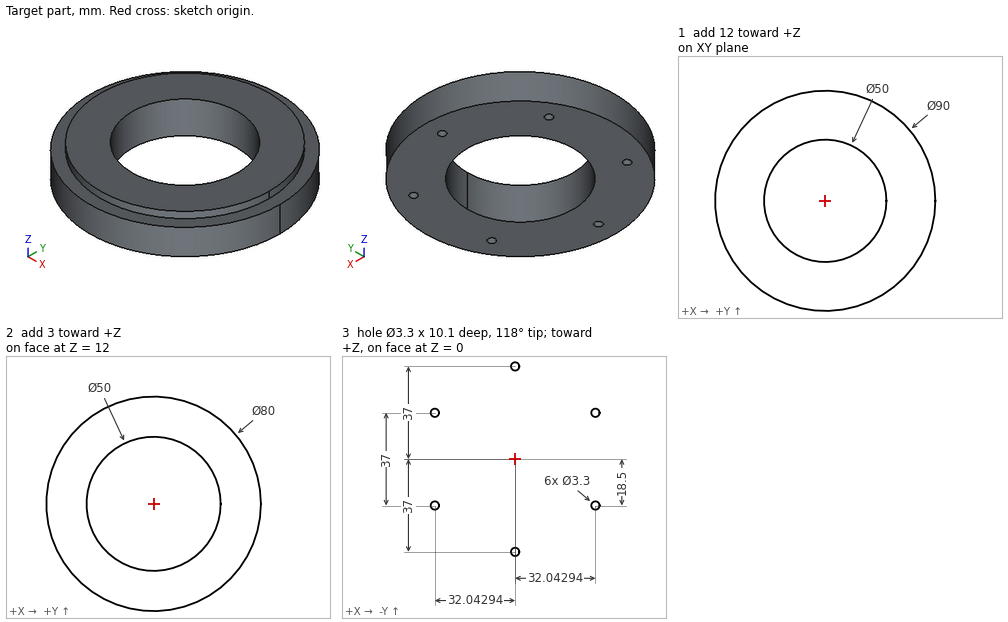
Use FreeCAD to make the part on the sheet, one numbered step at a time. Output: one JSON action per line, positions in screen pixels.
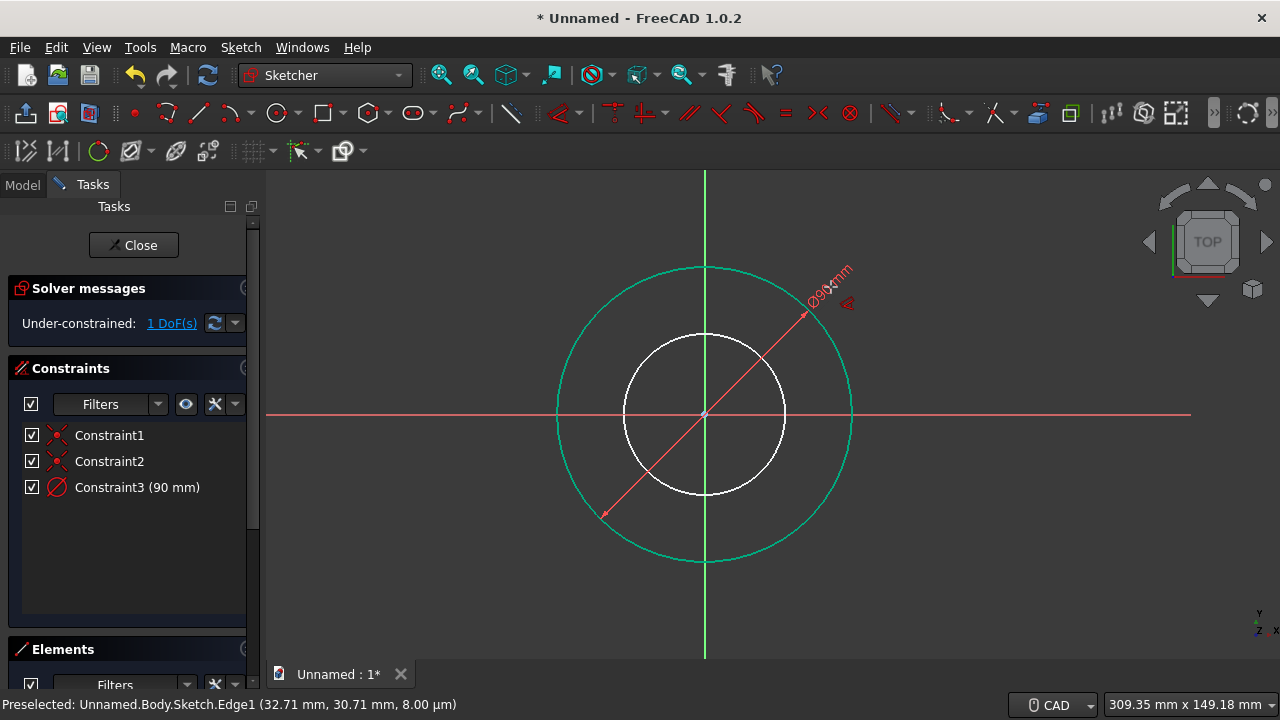
{"action": "left_click", "coordinate": [761, 357]}
{"action": "left_click", "coordinate": [783, 334]}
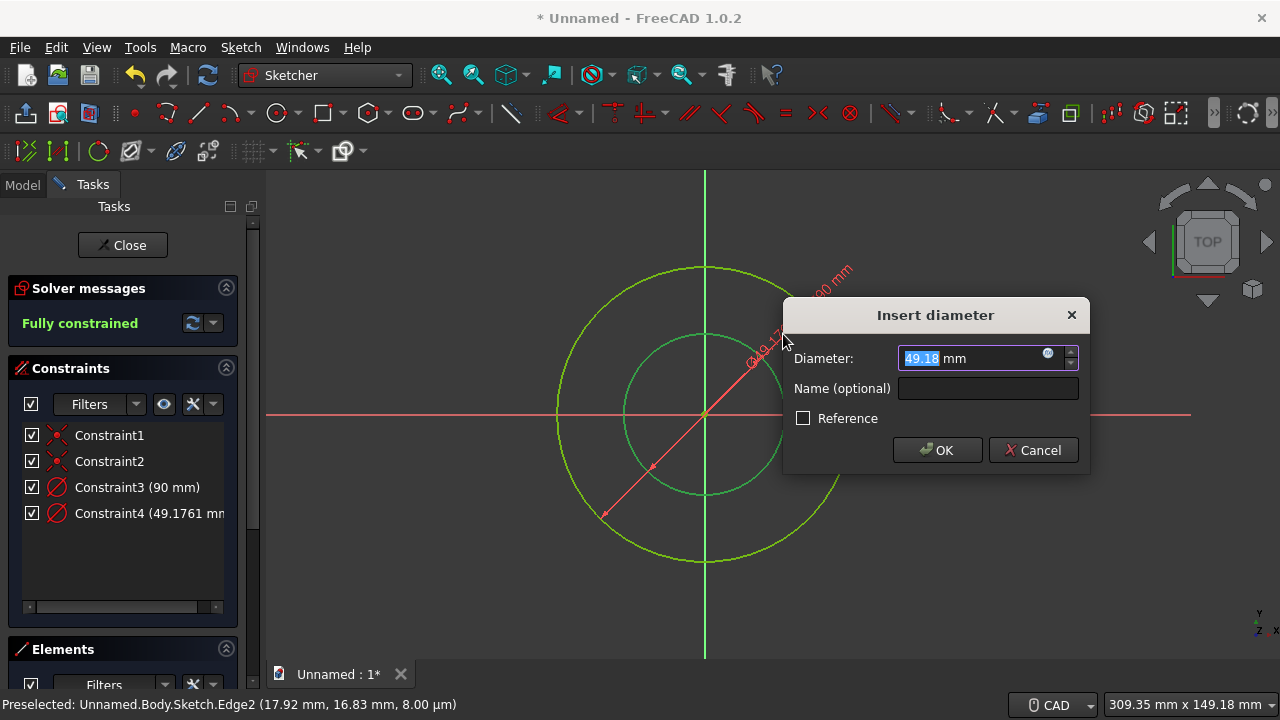
{"action": "type", "text": "50"}
{"action": "key", "text": "Return"}
{"action": "key", "text": "Escape"}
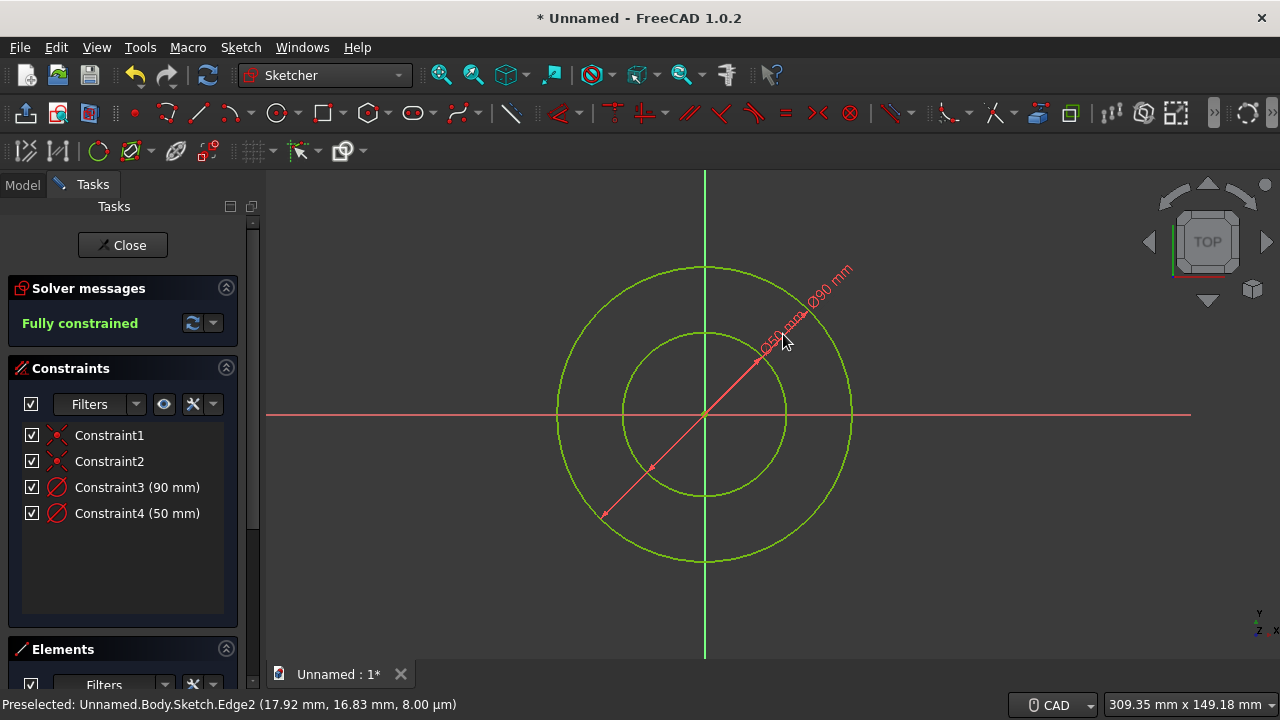
{"action": "left_click", "coordinate": [123, 245]}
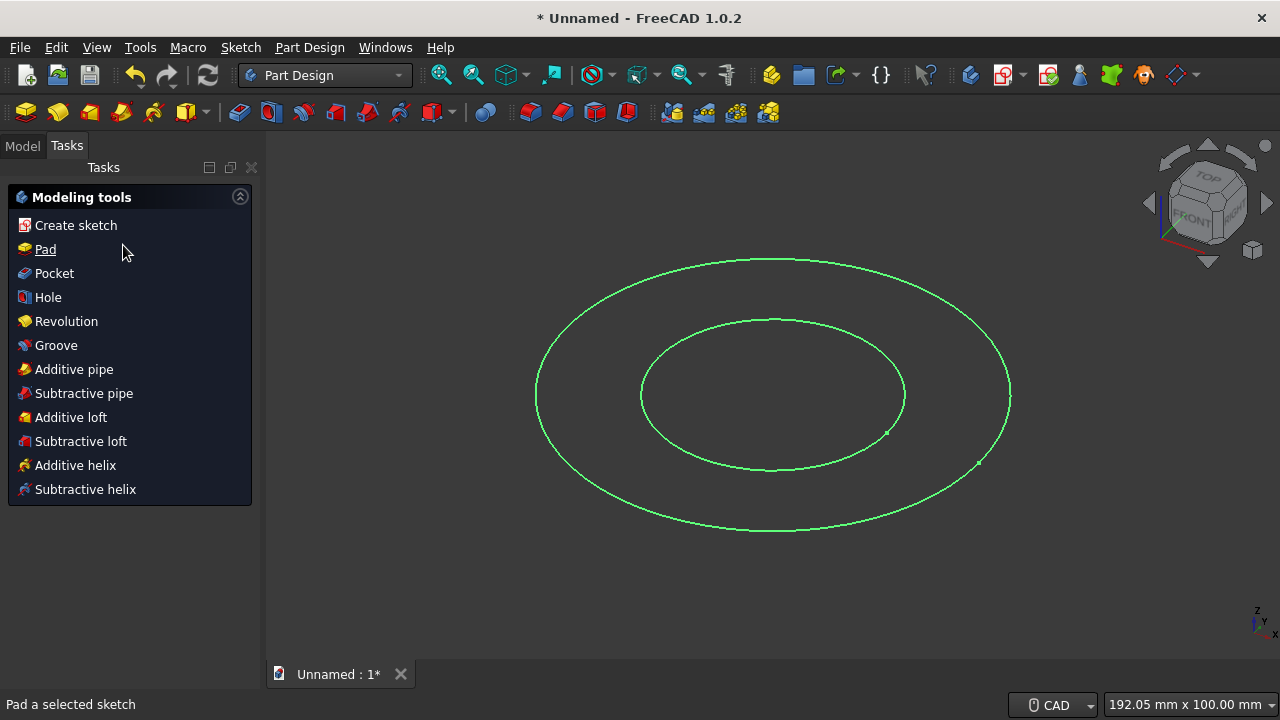
{"action": "left_click", "coordinate": [26, 112]}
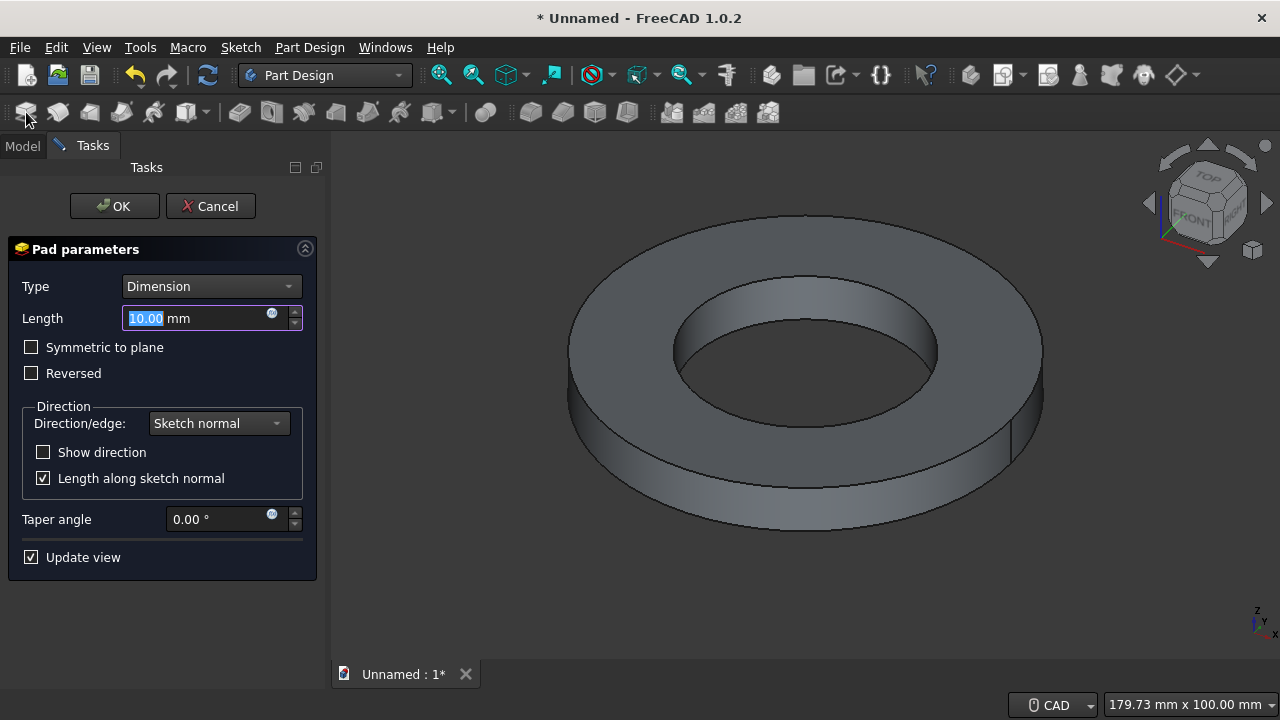
{"action": "type", "text": "12"}
{"action": "key", "text": "Tab"}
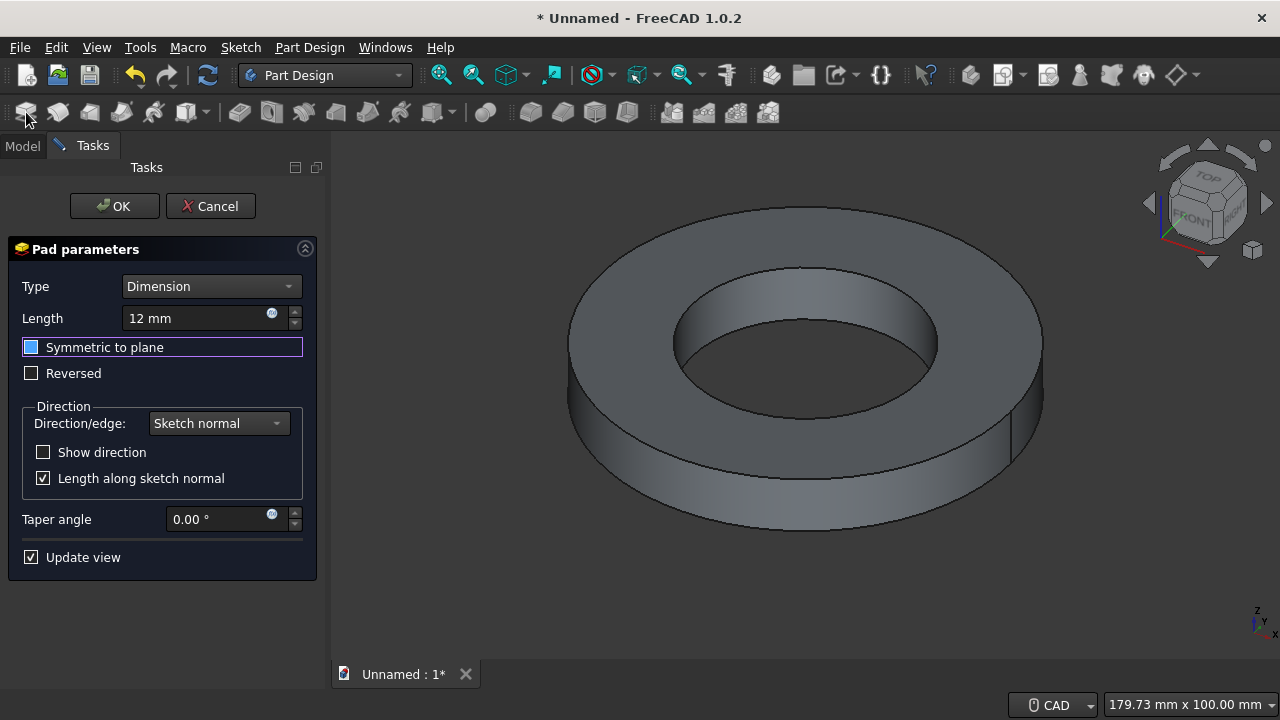
{"action": "left_click", "coordinate": [115, 206]}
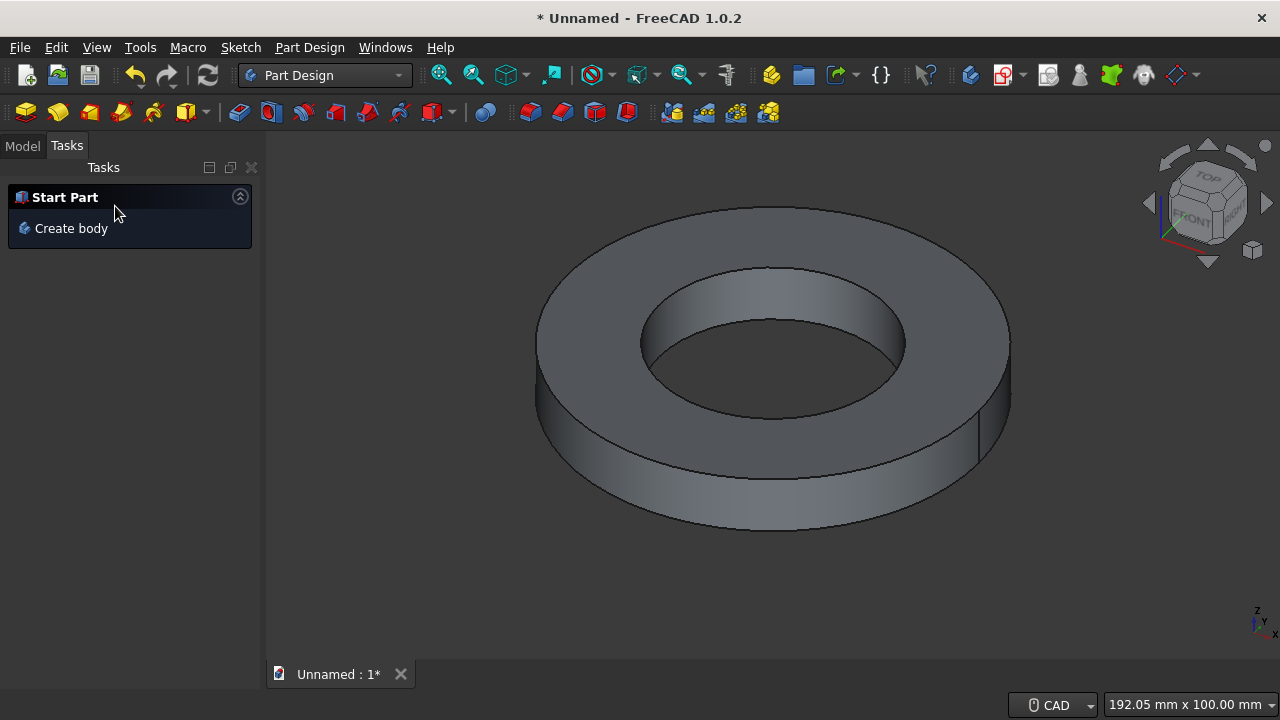
{"action": "left_click", "coordinate": [958, 314]}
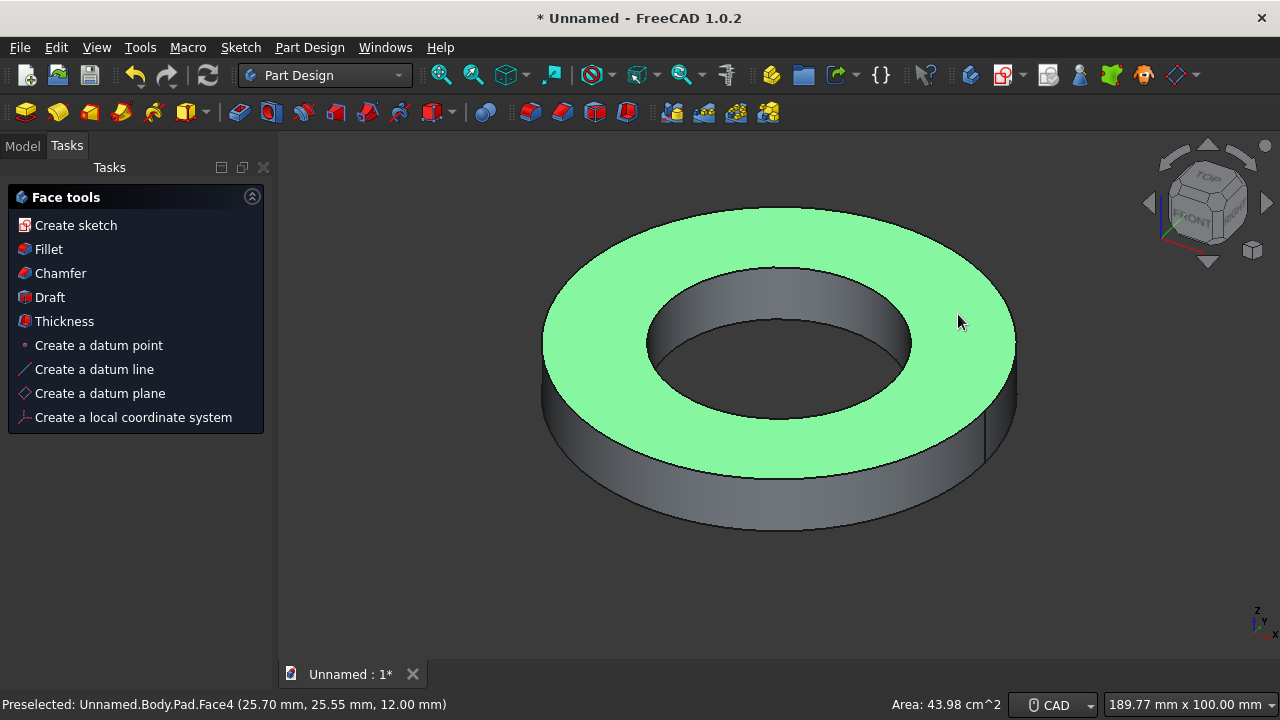
{"action": "left_click", "coordinate": [1004, 76]}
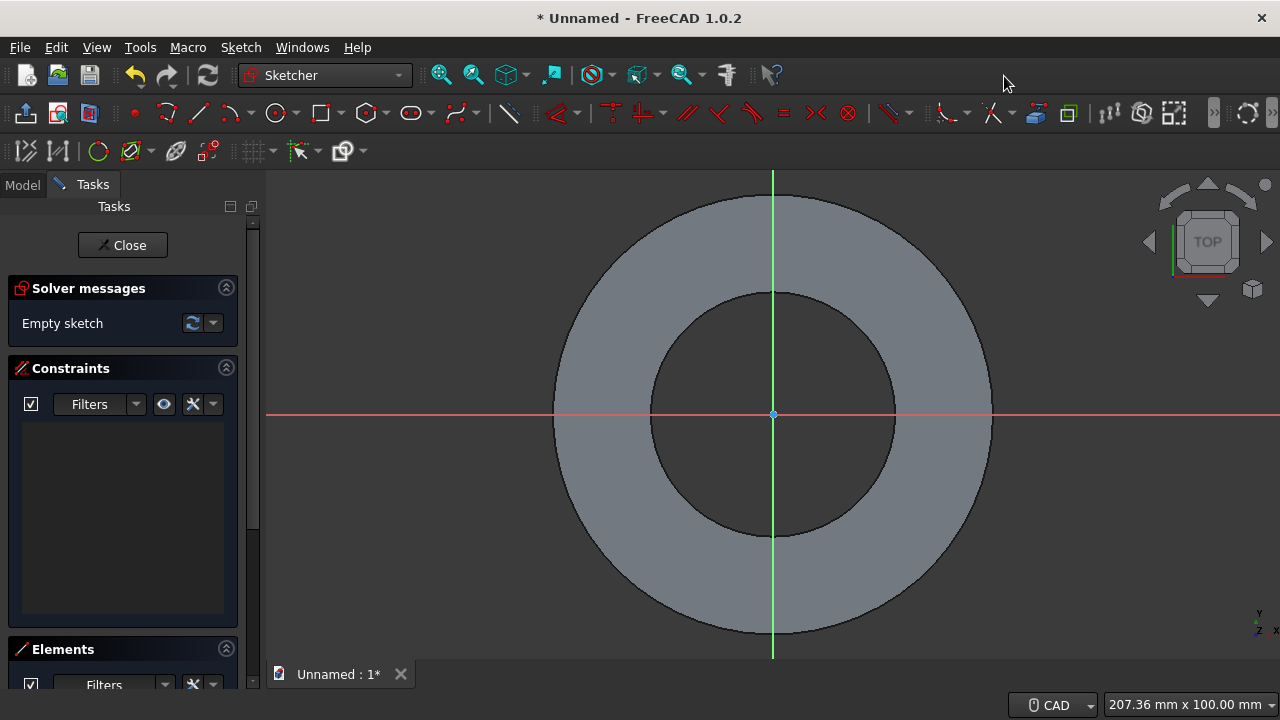
{"action": "scroll", "coordinate": [395, 415], "scroll_direction": "down", "scroll_amount": 1}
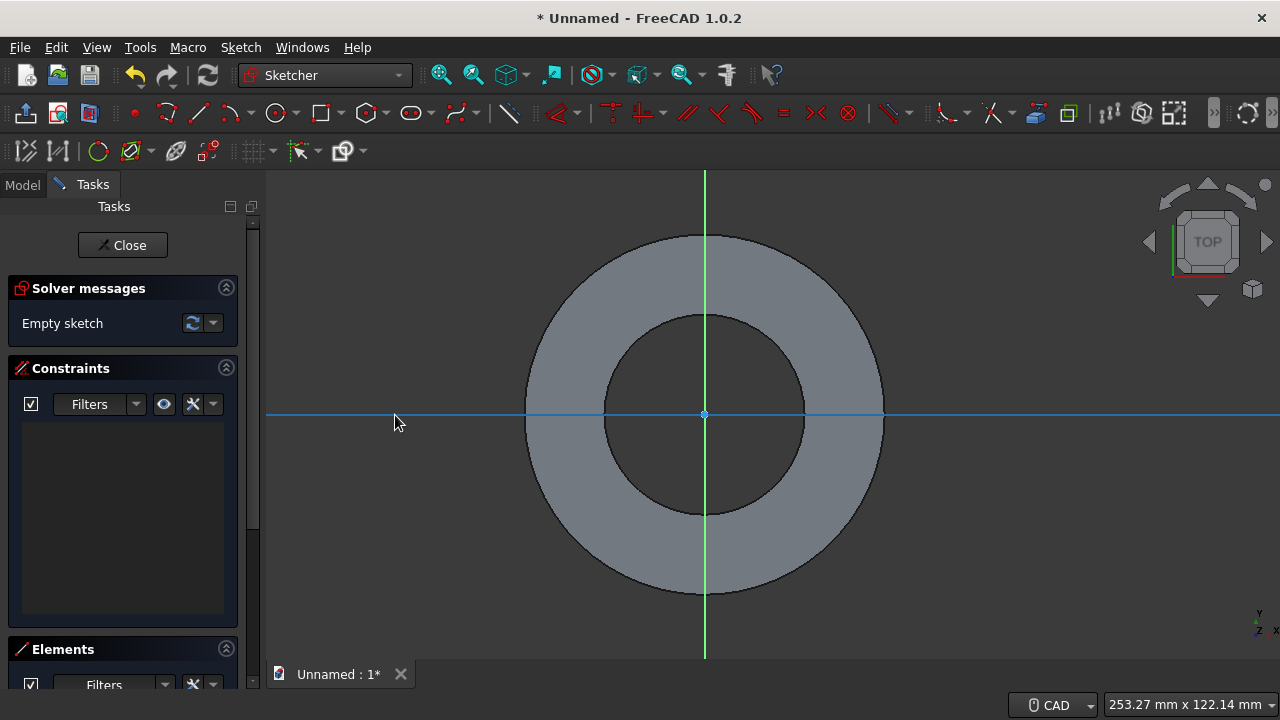
{"action": "left_click", "coordinate": [276, 114]}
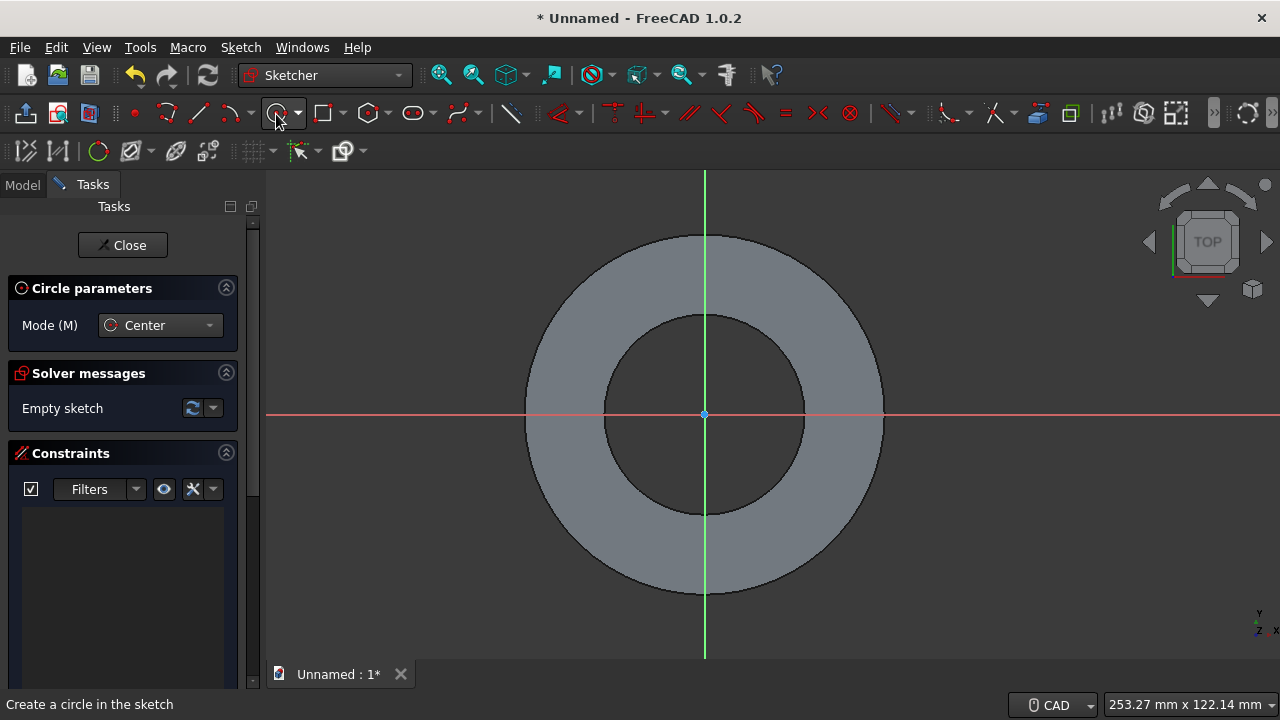
{"action": "left_click", "coordinate": [705, 415]}
{"action": "left_click", "coordinate": [818, 301]}